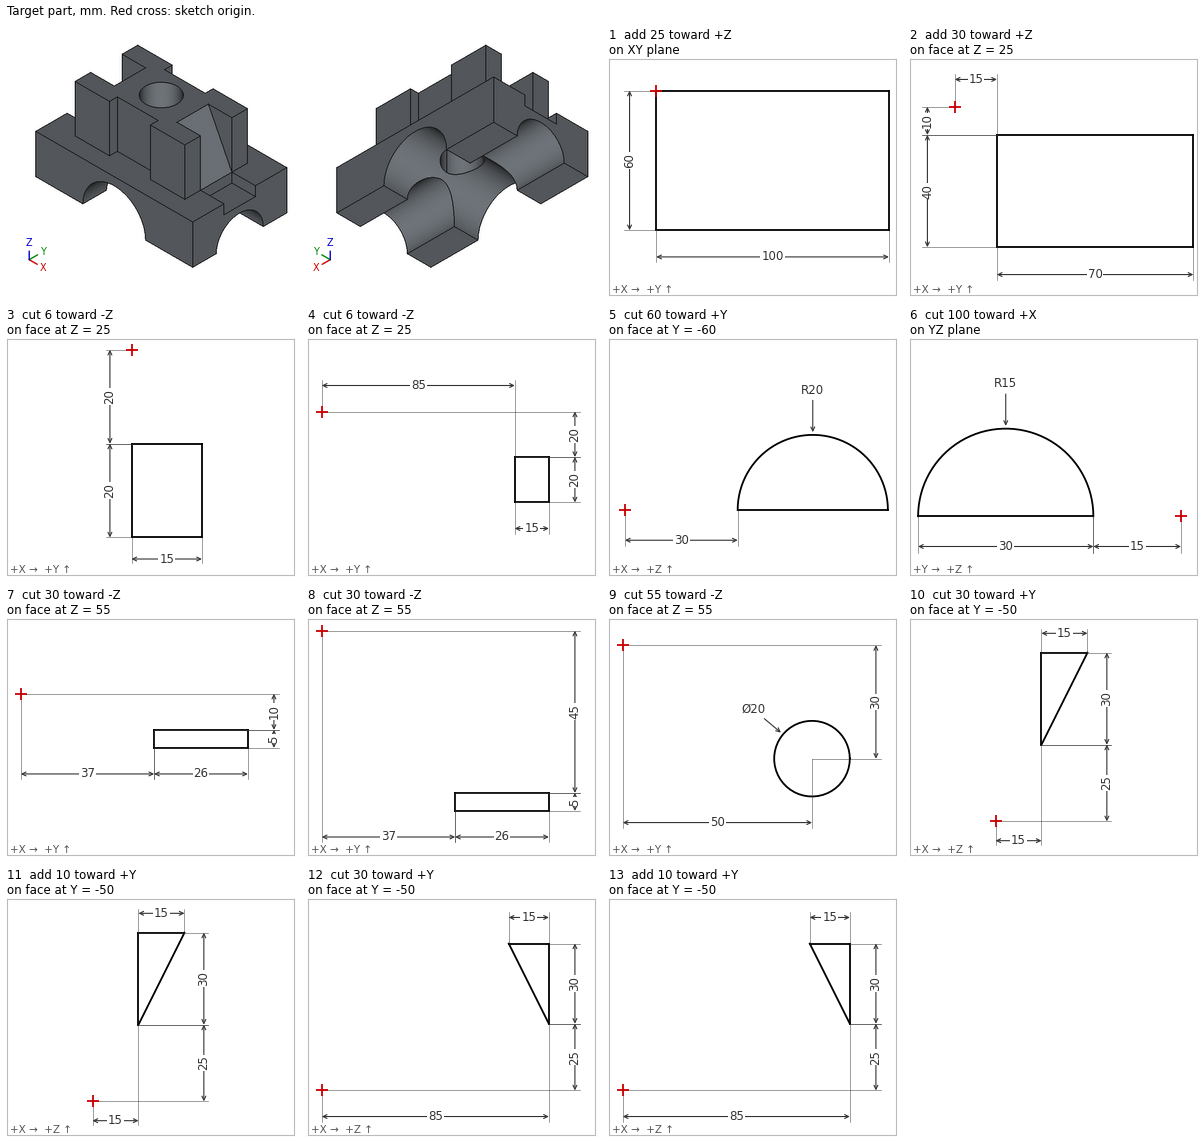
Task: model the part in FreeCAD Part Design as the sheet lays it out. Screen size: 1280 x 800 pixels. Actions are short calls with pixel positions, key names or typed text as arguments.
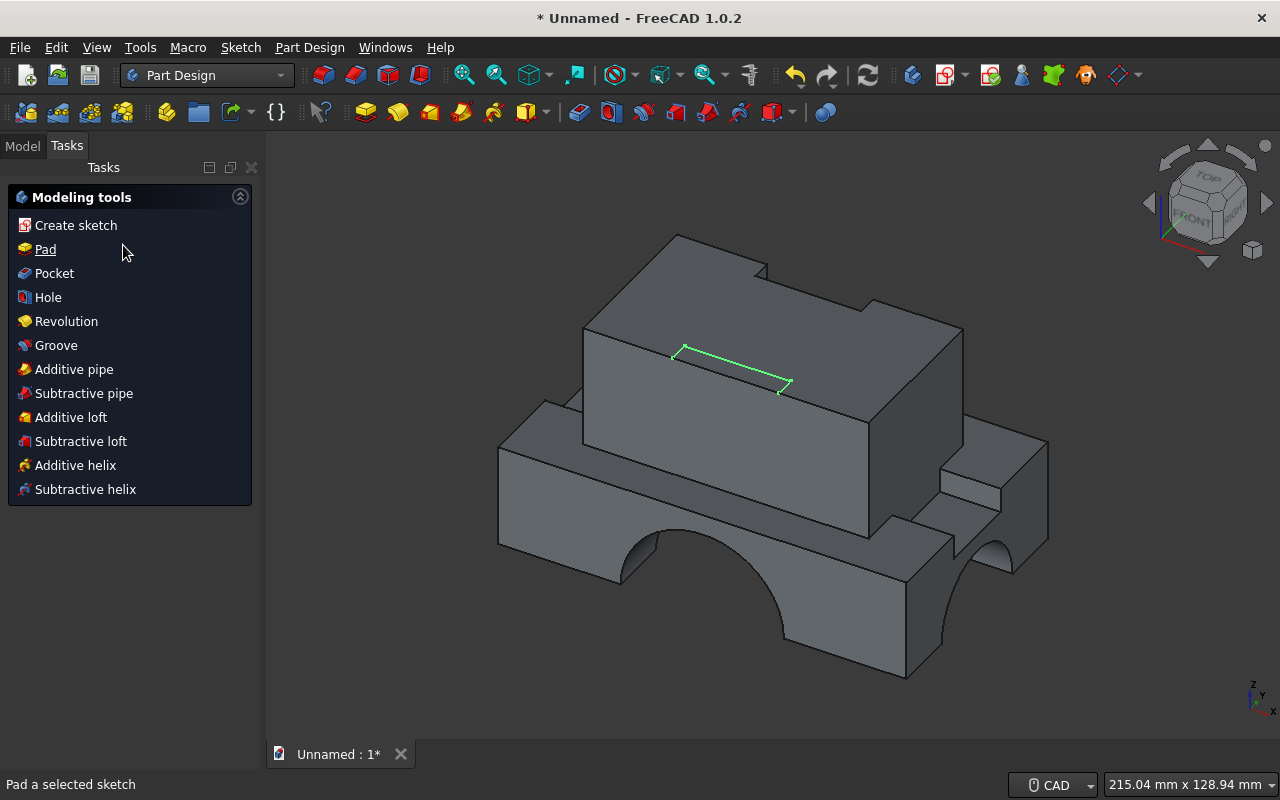
click(580, 112)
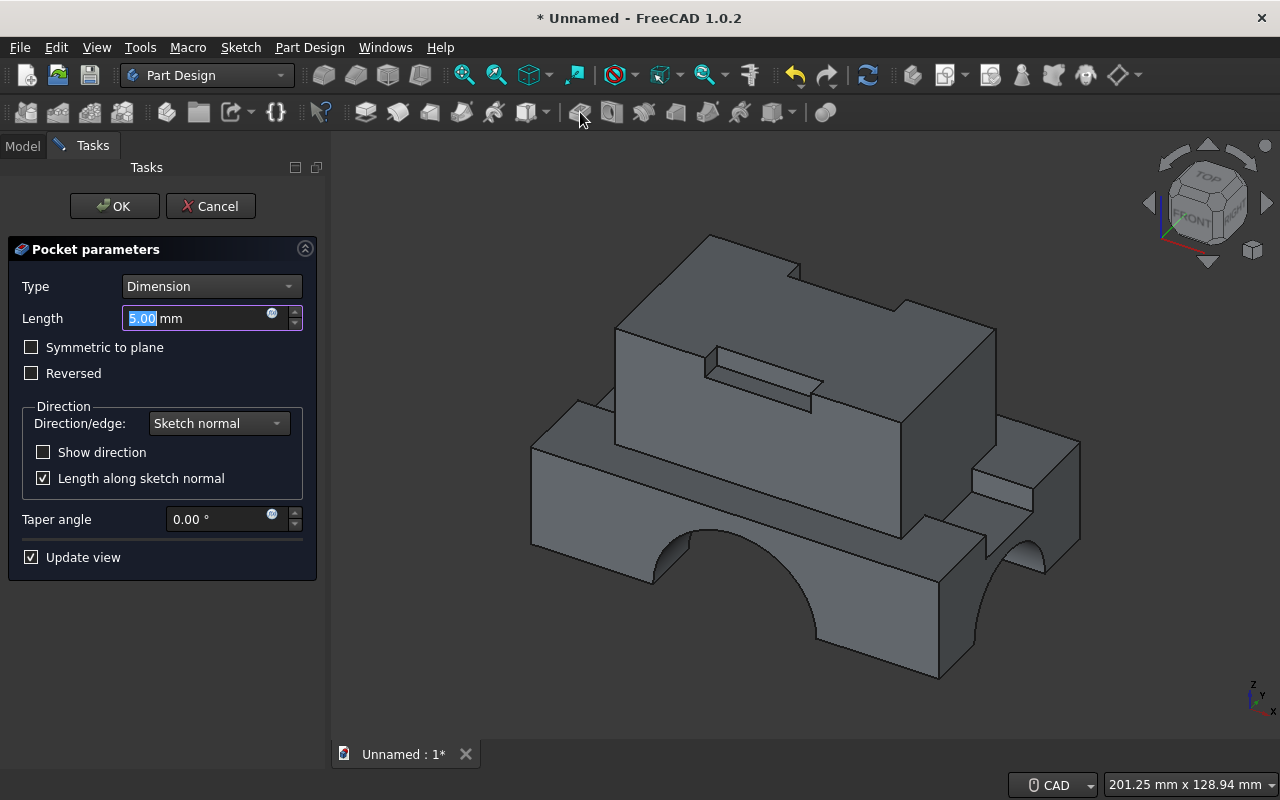
text(30)
key(Tab)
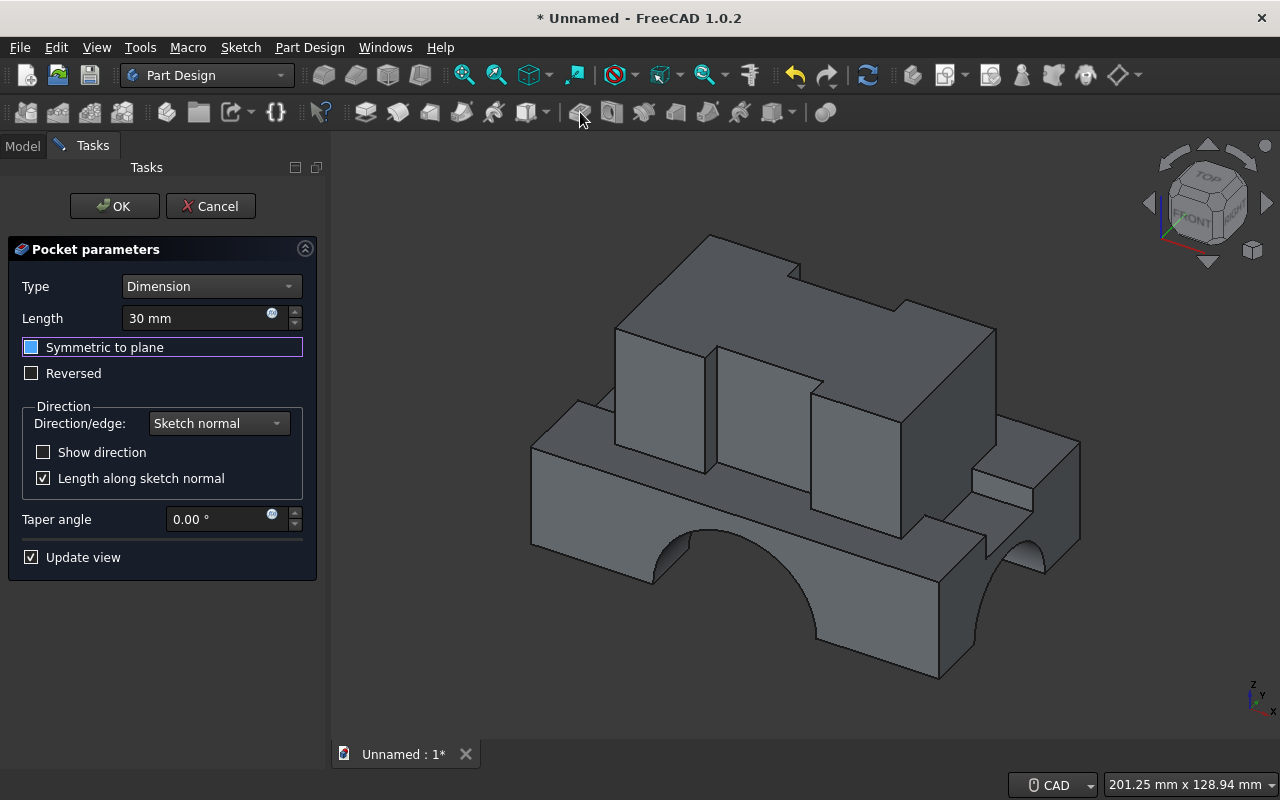
click(115, 206)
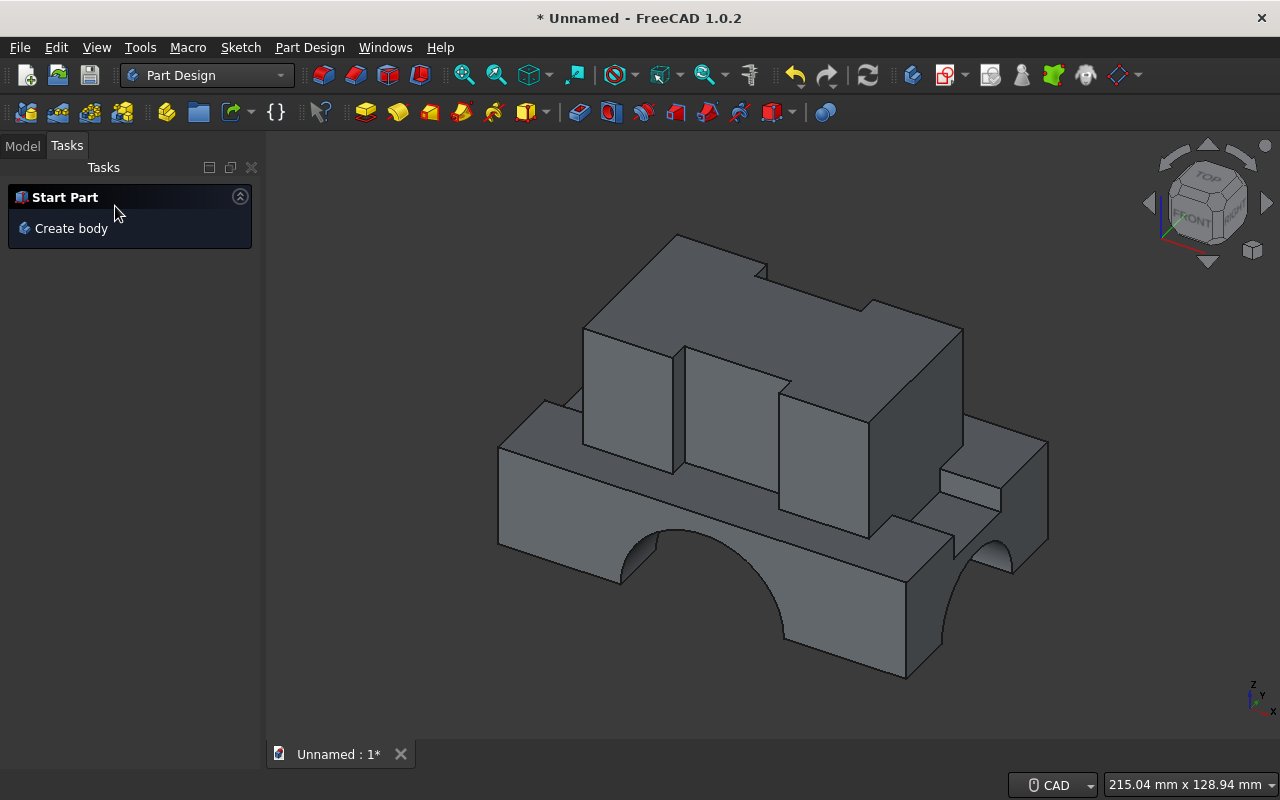
click(855, 355)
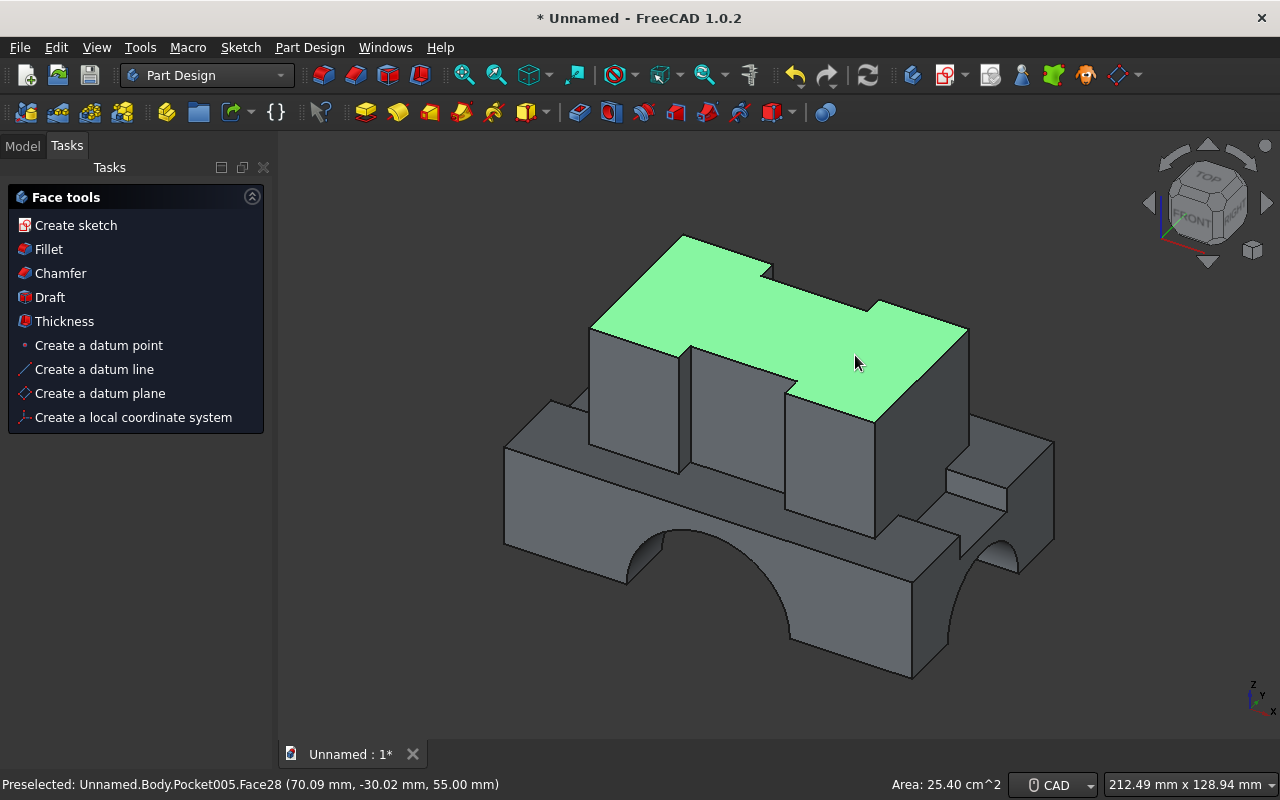
click(946, 76)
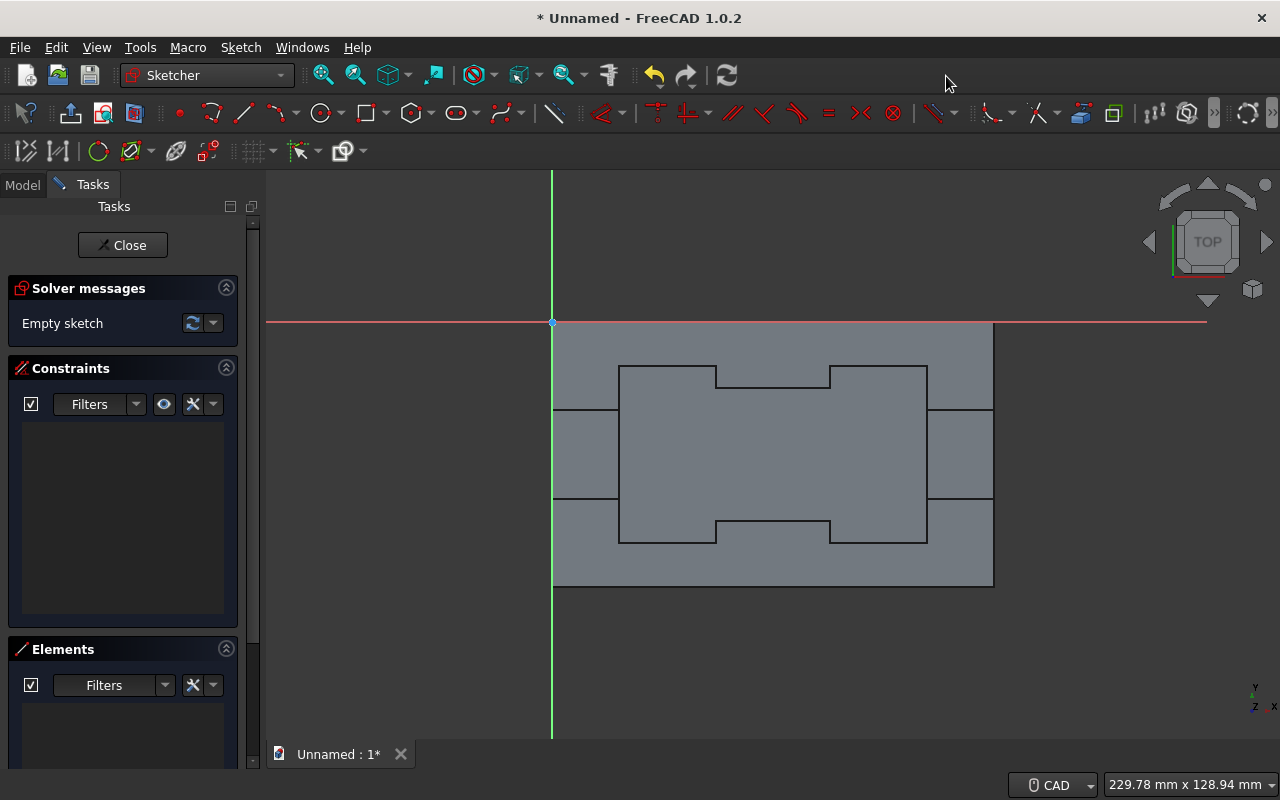
scroll(795, 454, up, 7)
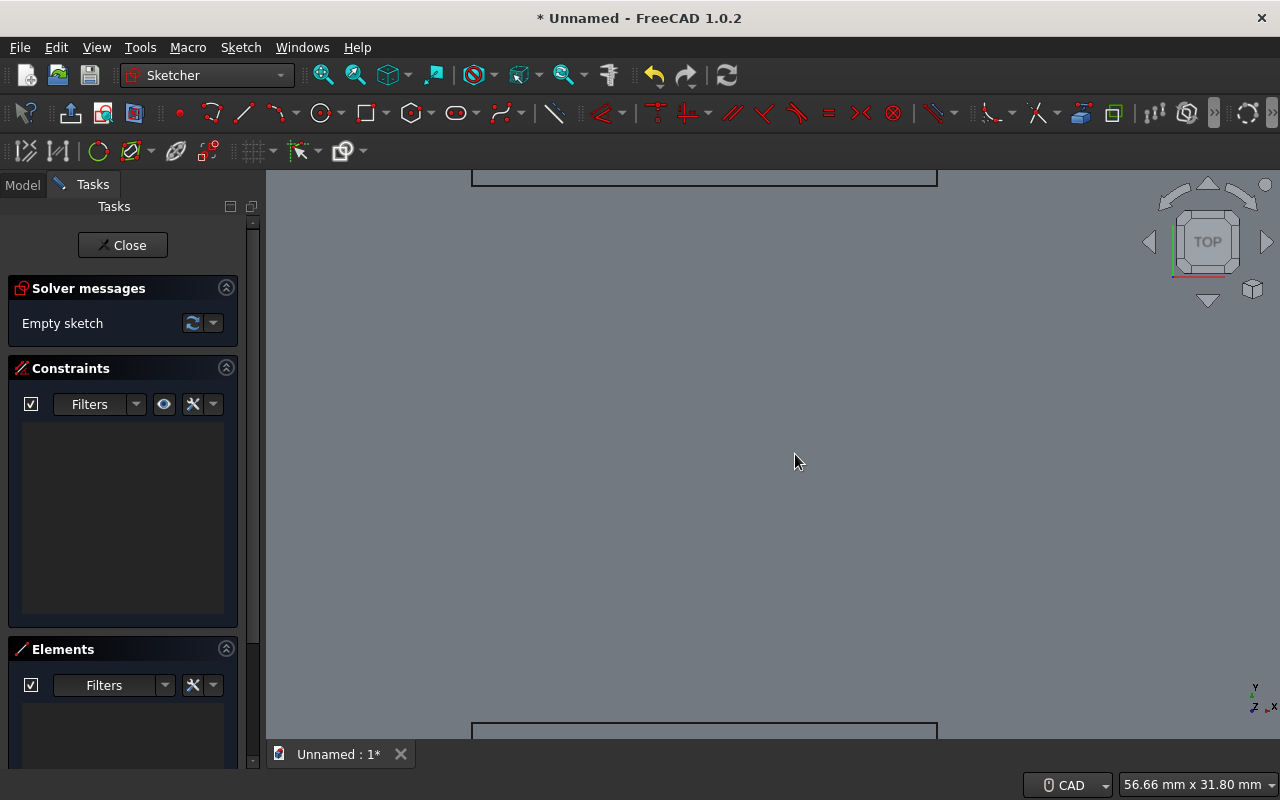
key(g)
key(c)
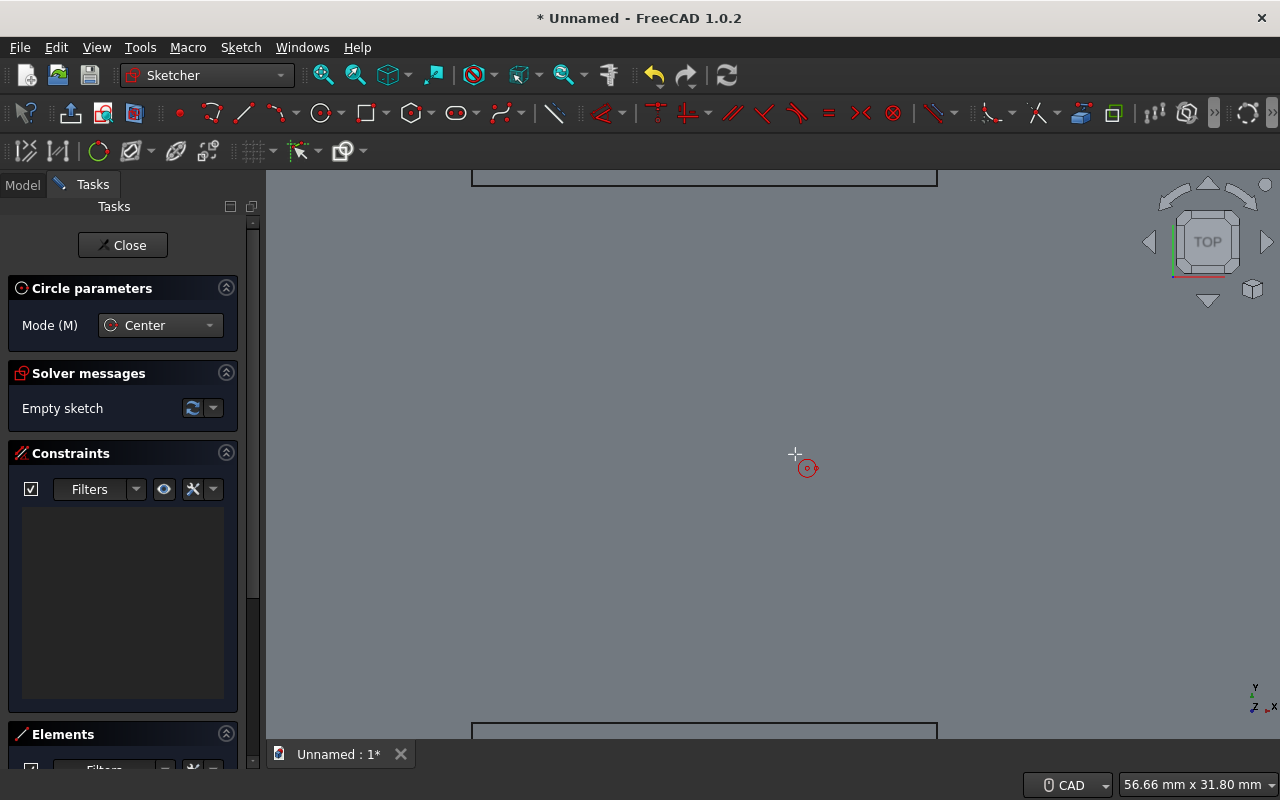
click(704, 454)
click(831, 328)
key(Escape)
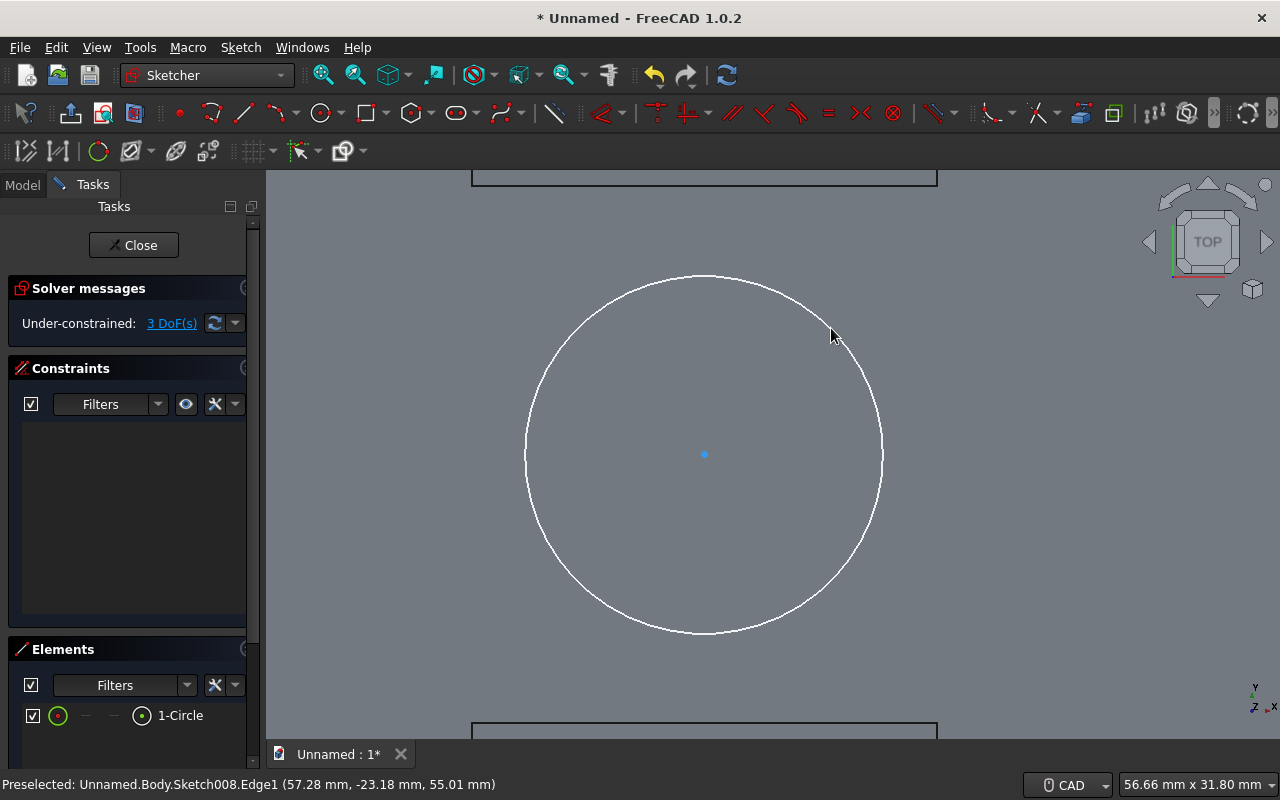
click(602, 114)